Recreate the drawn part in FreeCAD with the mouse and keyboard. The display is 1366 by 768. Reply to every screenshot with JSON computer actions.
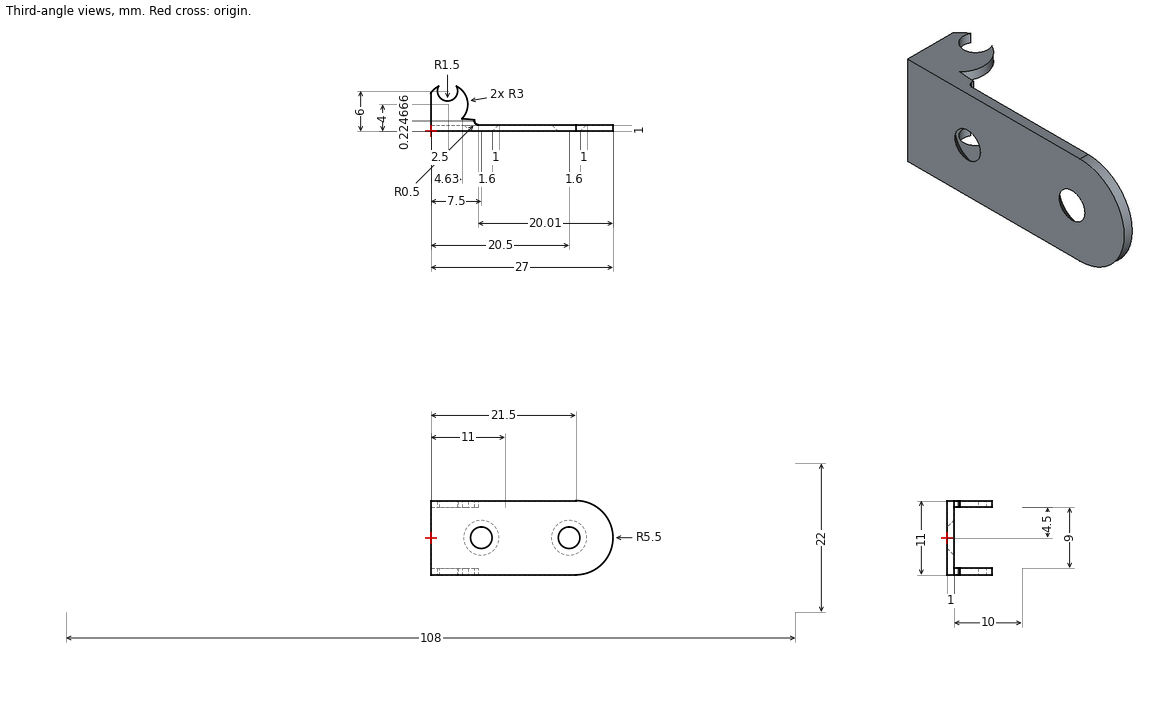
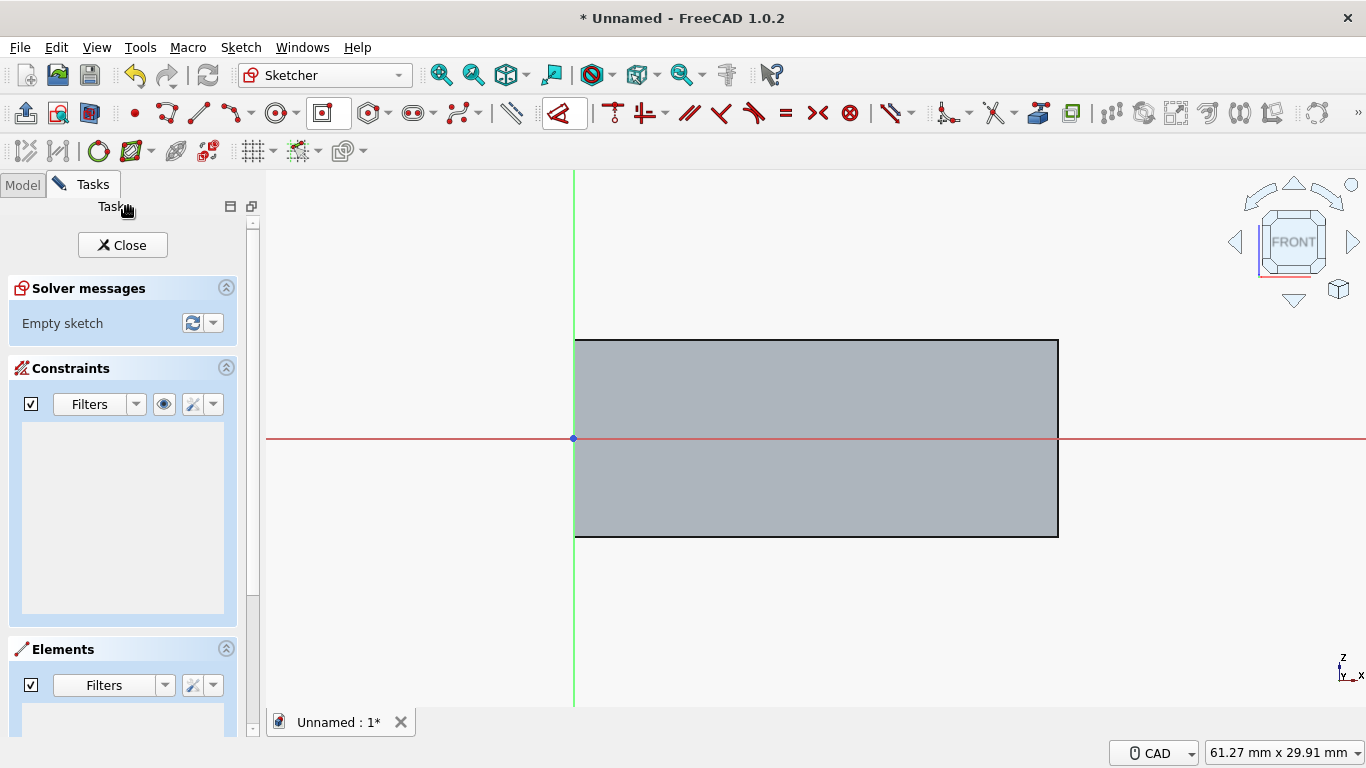
{"action": "scroll", "coordinate": [822, 438], "scroll_direction": "down", "scroll_amount": 6}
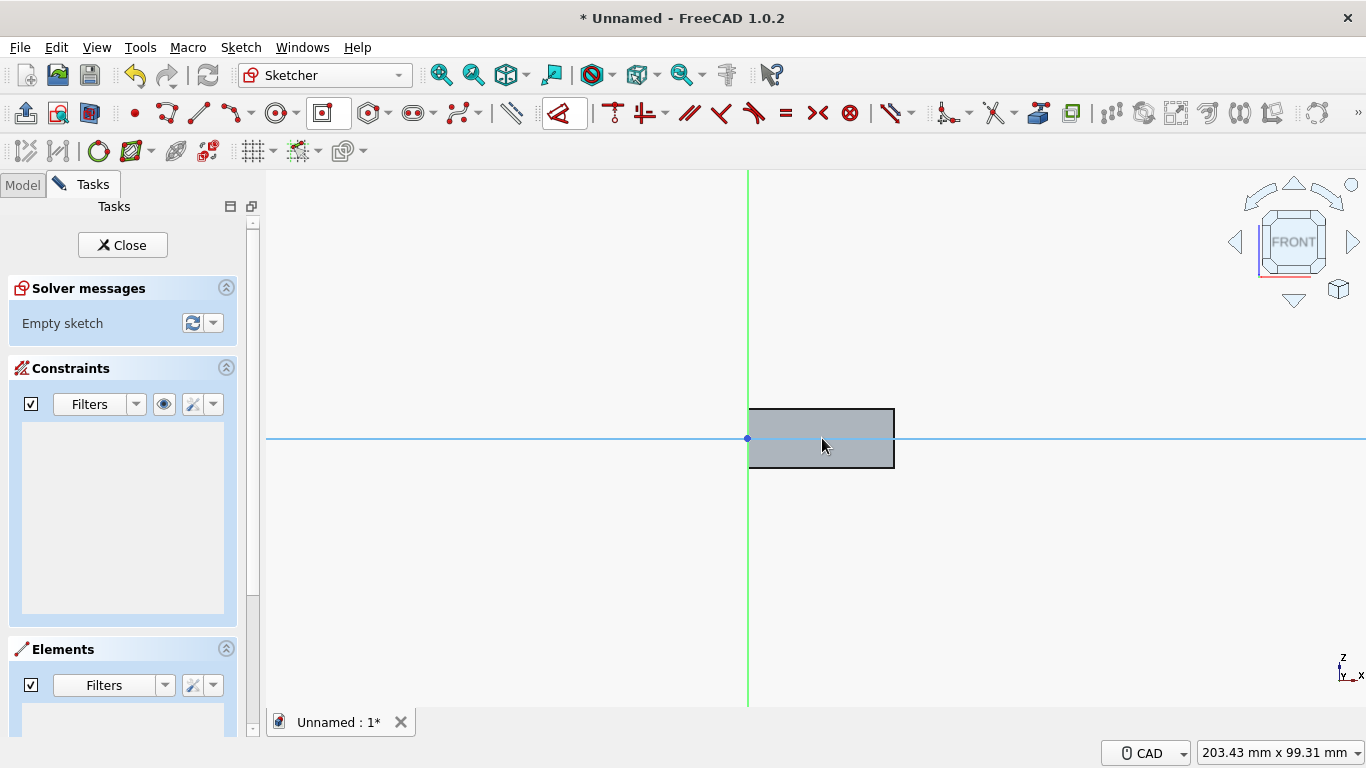
{"action": "key", "text": "g v"}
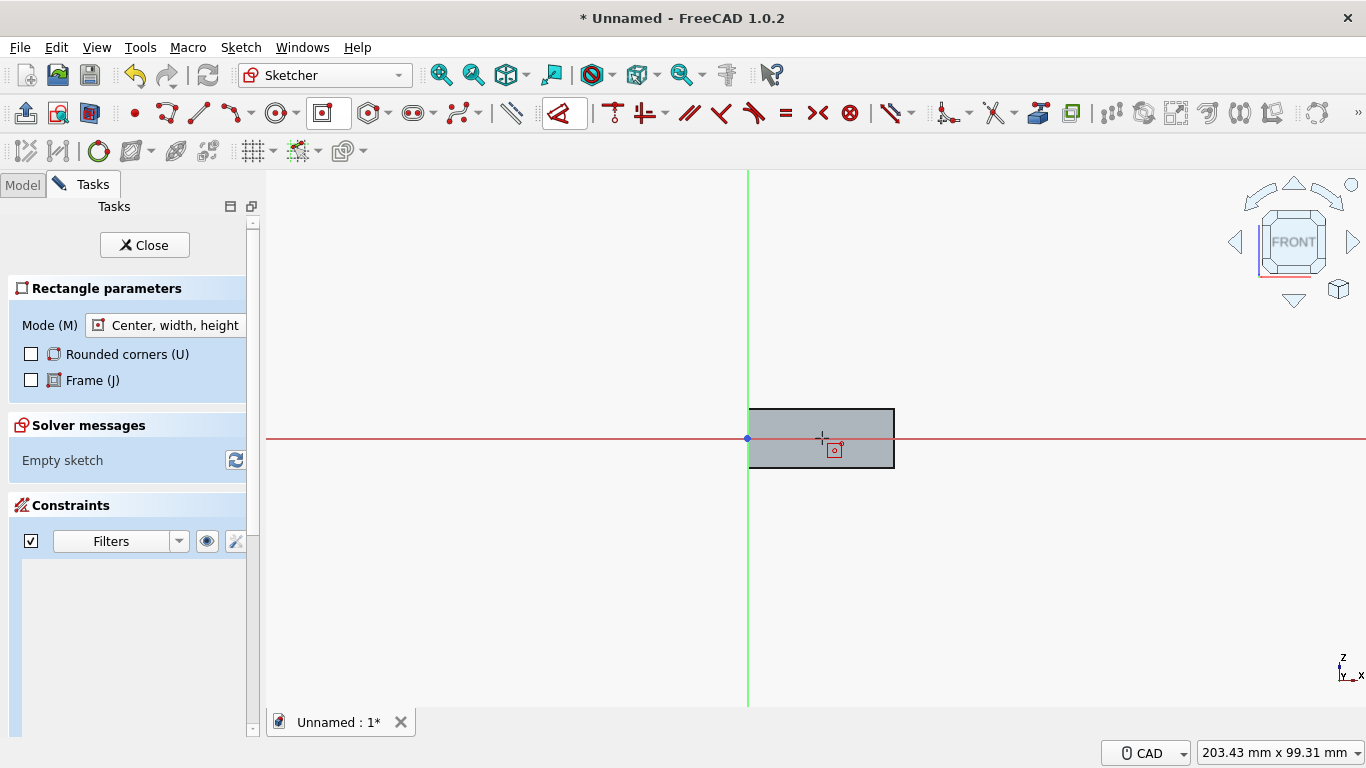
{"action": "left_click", "coordinate": [748, 439]}
{"action": "left_click", "coordinate": [1040, 379]}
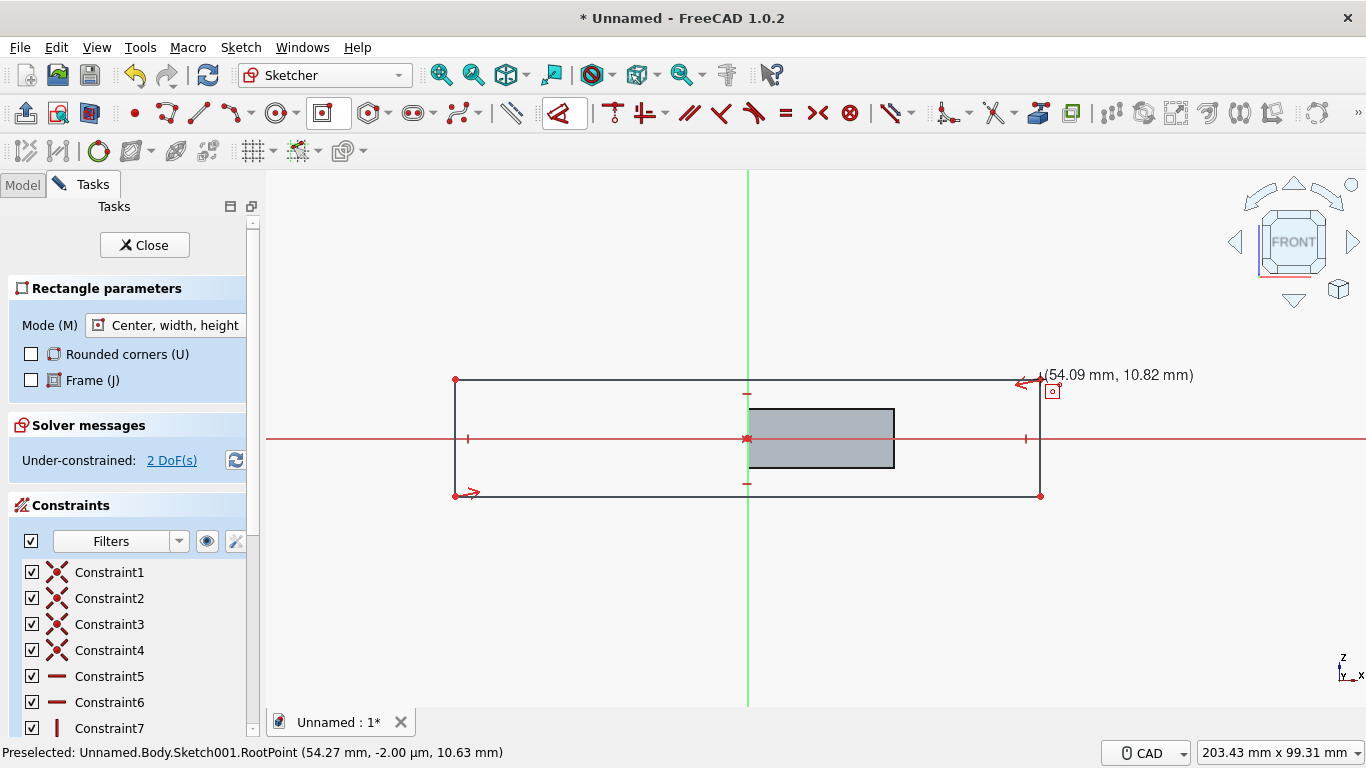
{"action": "key", "text": "g m"}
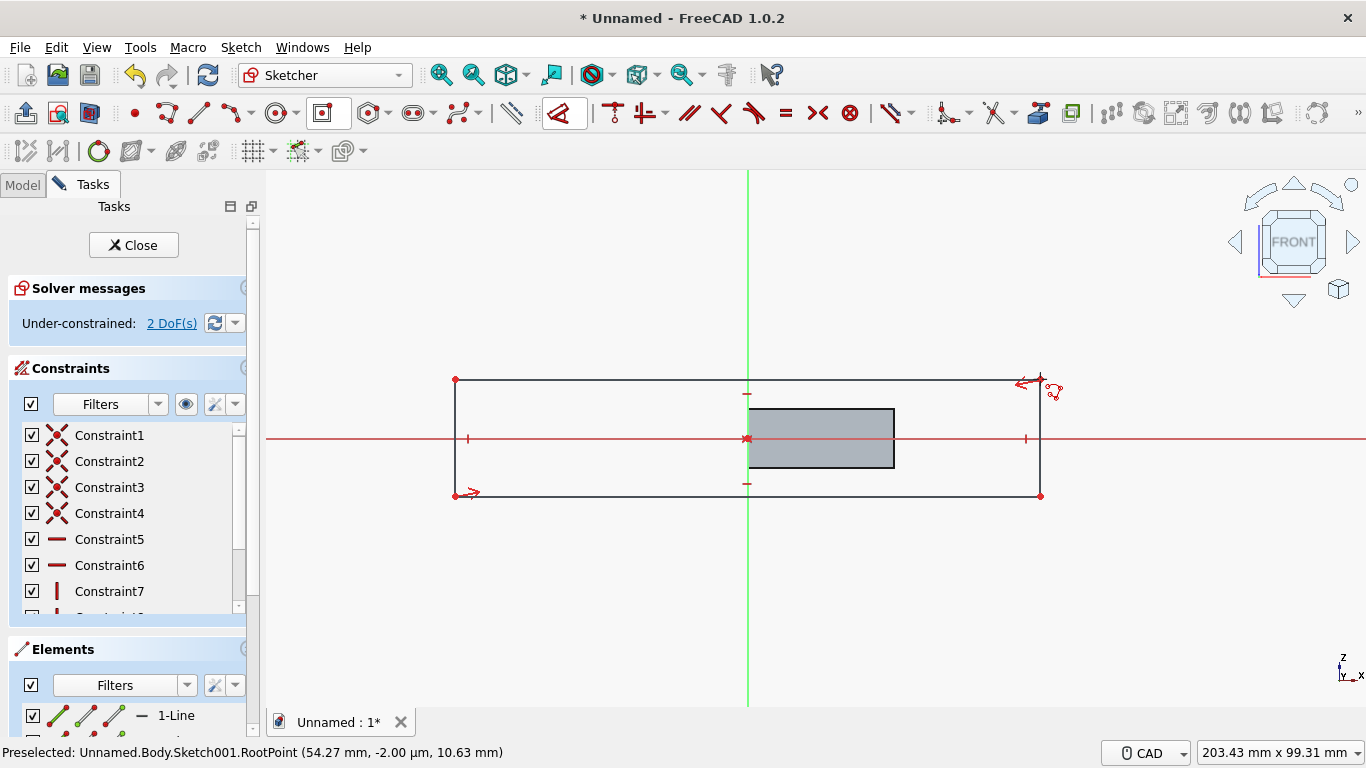
{"action": "left_click", "coordinate": [864, 409]}
{"action": "left_click", "coordinate": [748, 409]}
{"action": "left_click", "coordinate": [757, 468]}
{"action": "left_click", "coordinate": [864, 468]}
{"action": "right_click", "coordinate": [864, 468]}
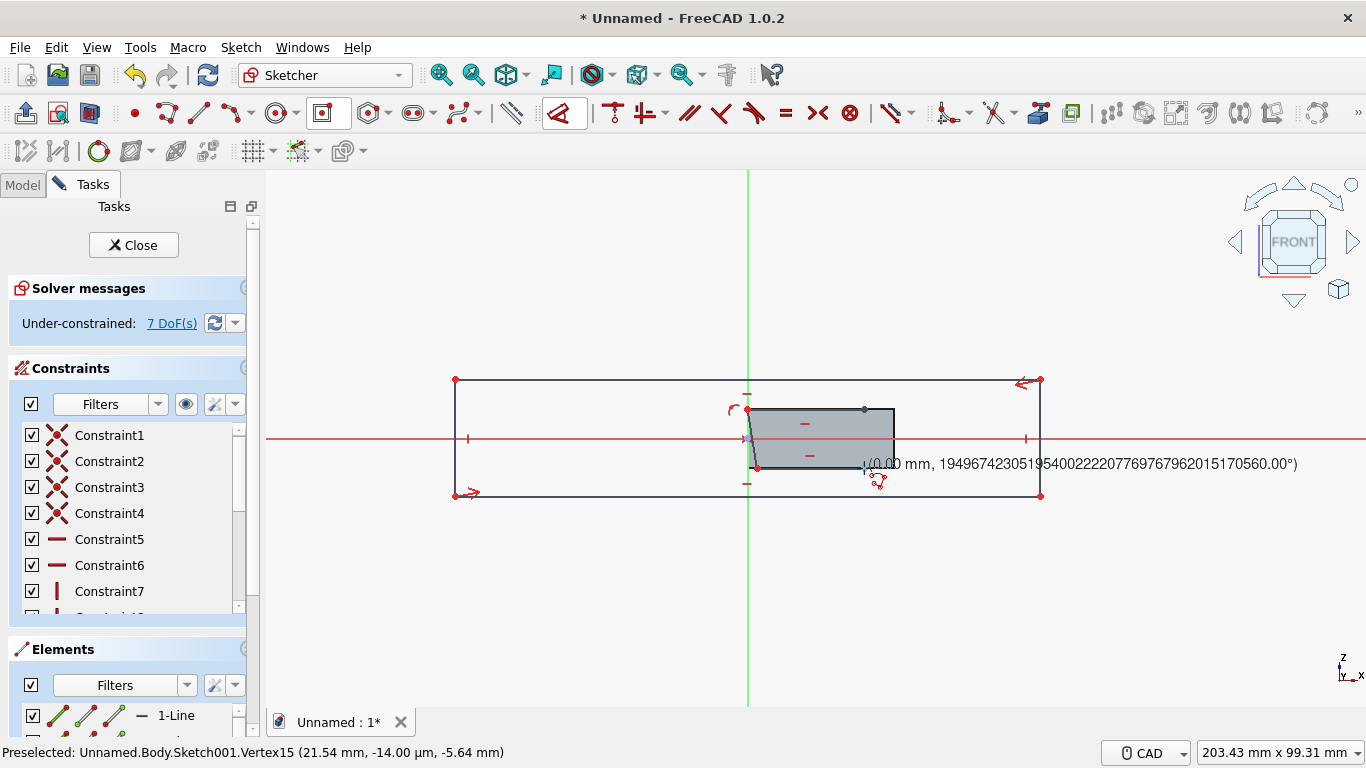
{"action": "left_click", "coordinate": [232, 114]}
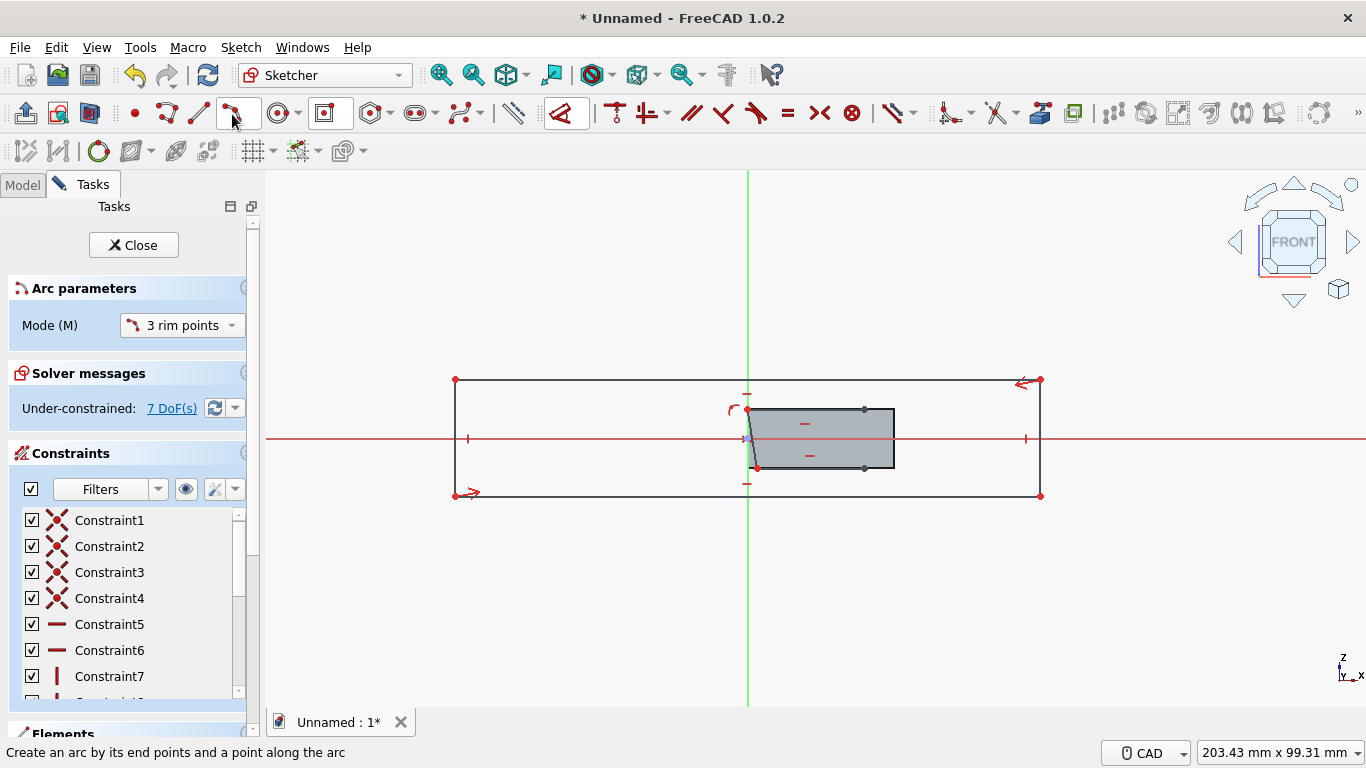
{"action": "left_click", "coordinate": [864, 469]}
{"action": "left_click", "coordinate": [864, 410]}
{"action": "left_click", "coordinate": [888, 456]}
{"action": "key", "text": "Escape"}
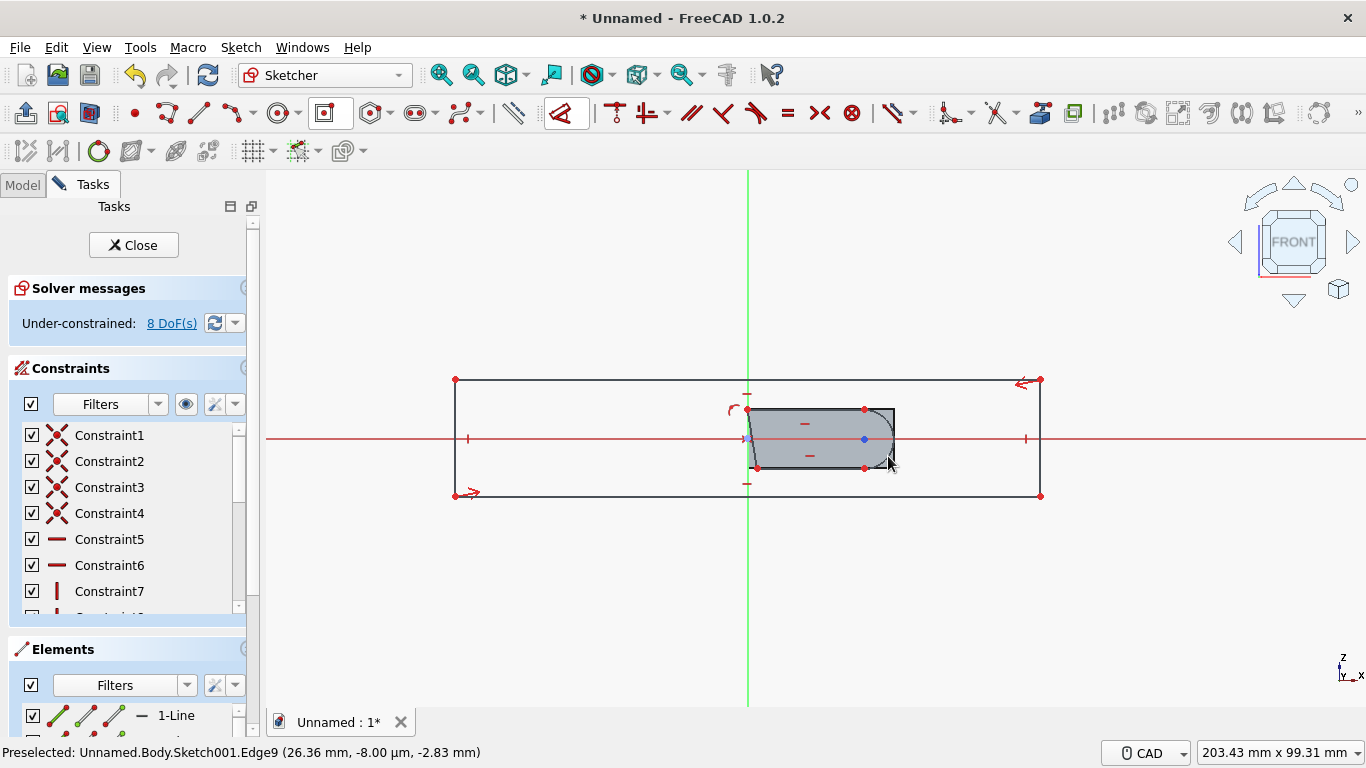
{"action": "left_click", "coordinate": [829, 410]}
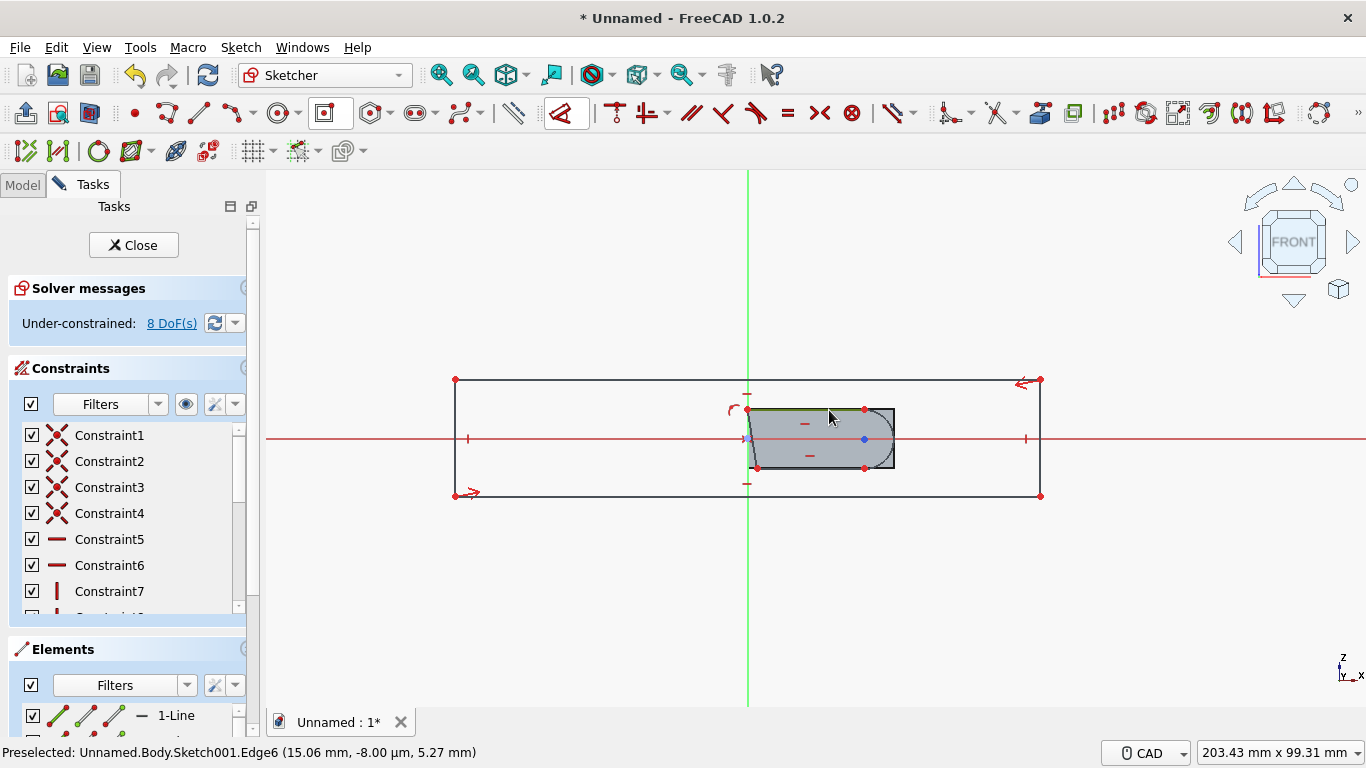
{"action": "left_click", "coordinate": [888, 457]}